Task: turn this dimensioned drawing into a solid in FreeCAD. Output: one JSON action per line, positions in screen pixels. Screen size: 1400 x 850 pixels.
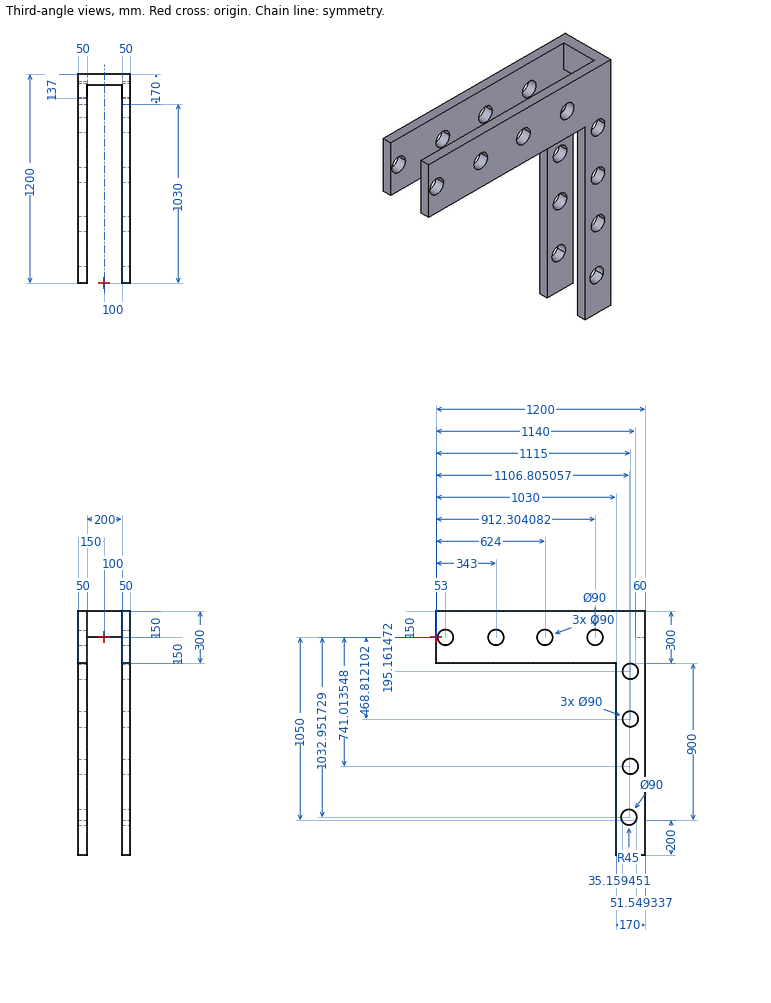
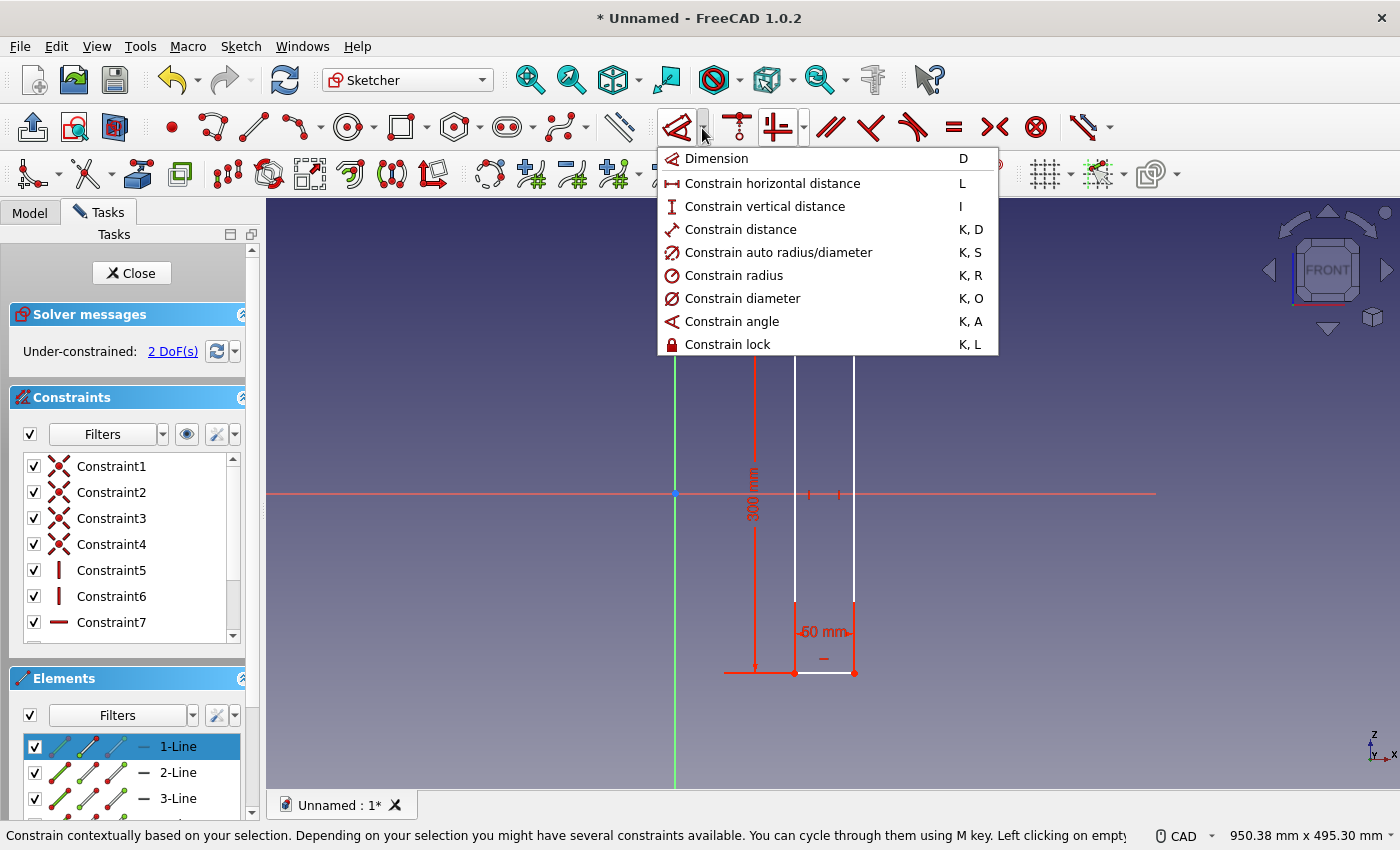
{"action": "left_click", "coordinate": [828, 184]}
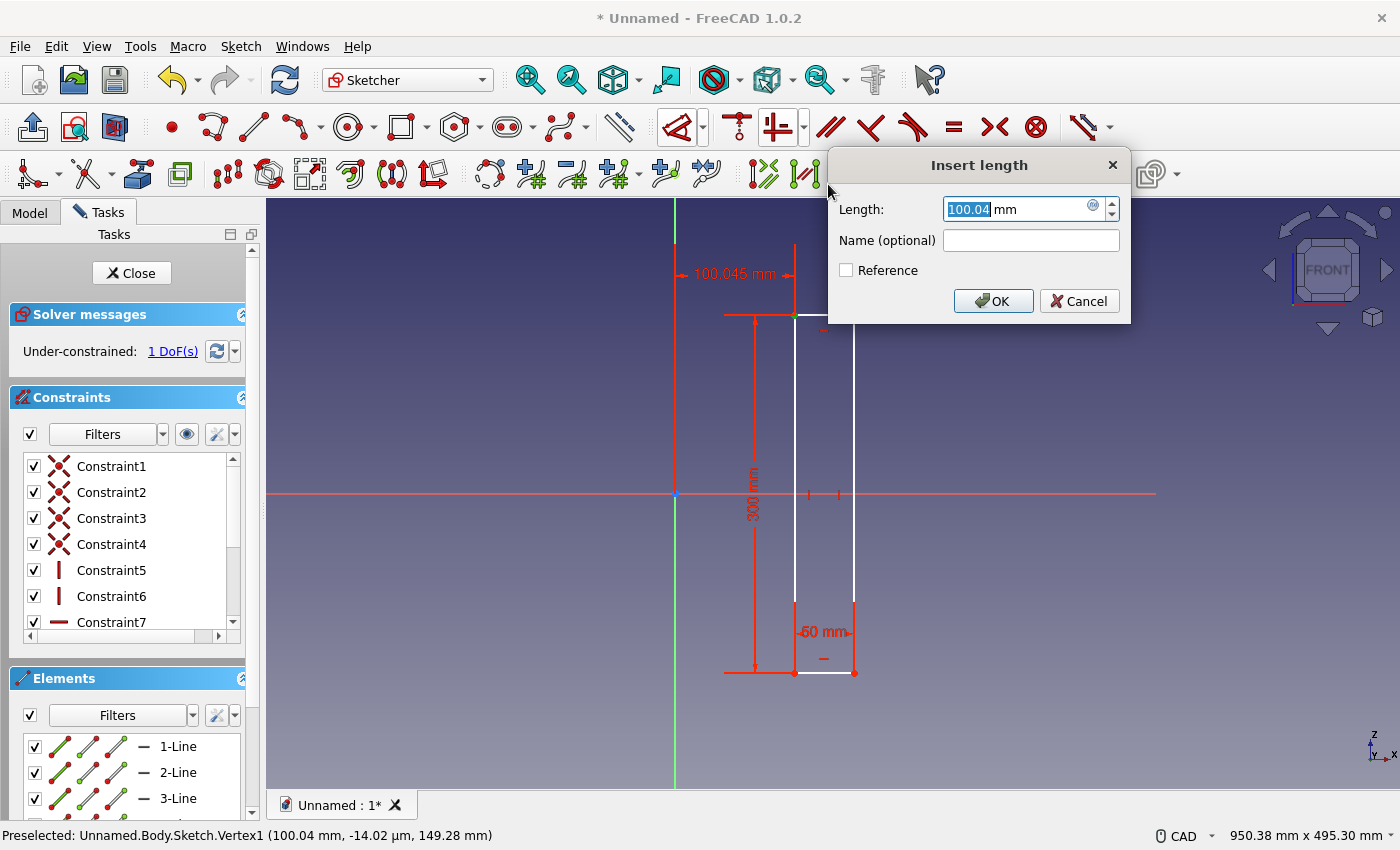
{"action": "type", "text": "100"}
{"action": "key", "text": "Return"}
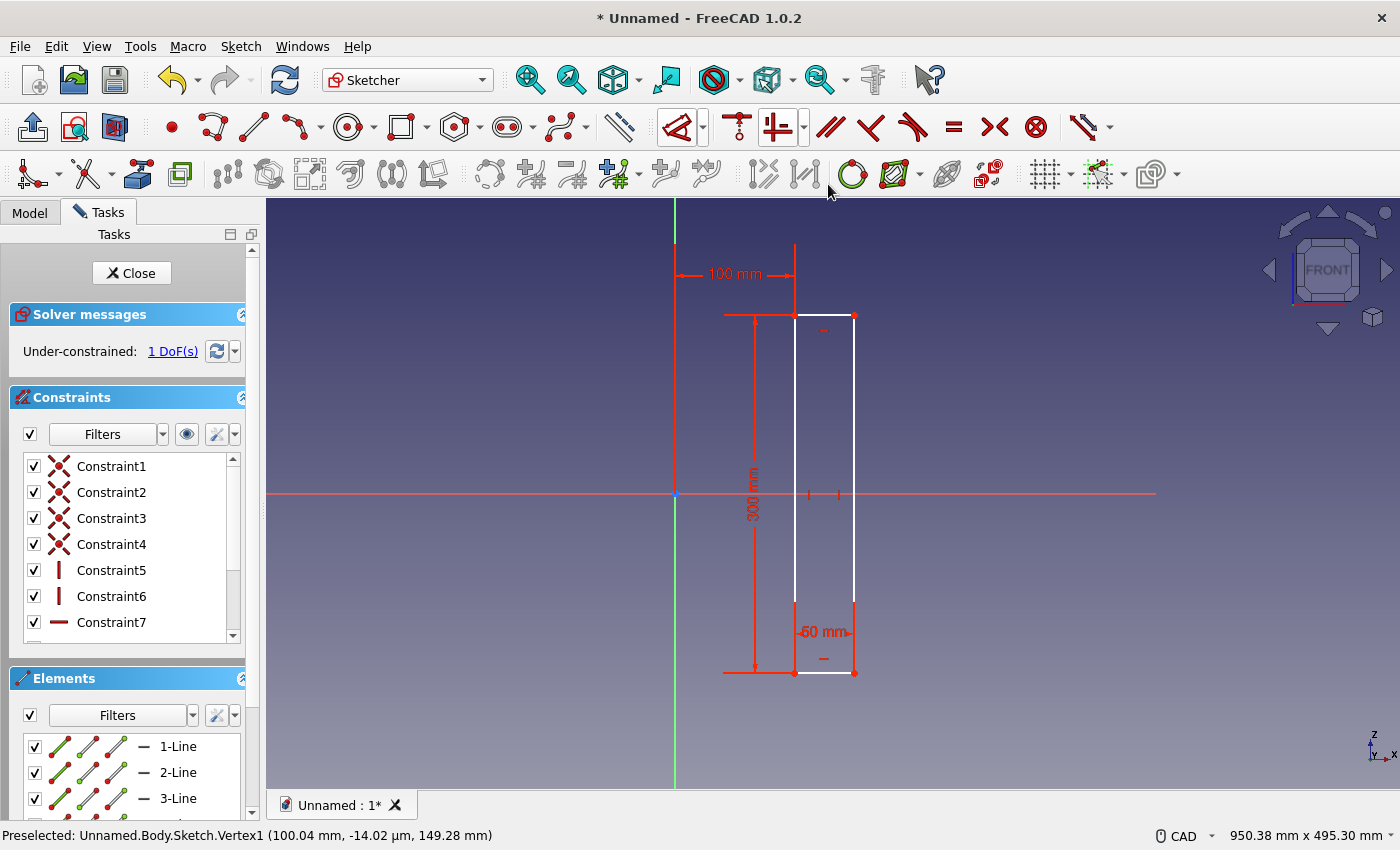
{"action": "left_click", "coordinate": [795, 315]}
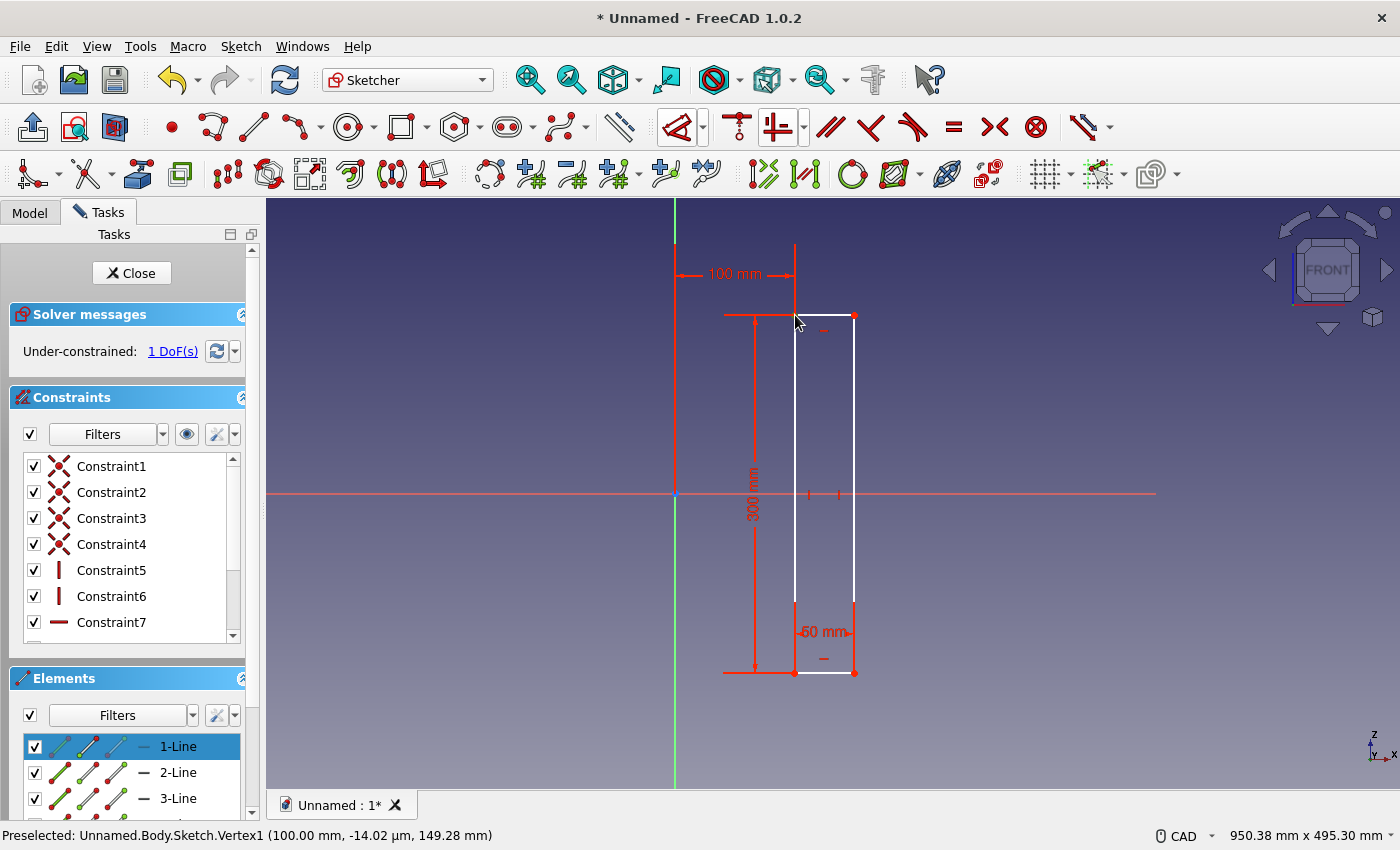
{"action": "key", "text": "i"}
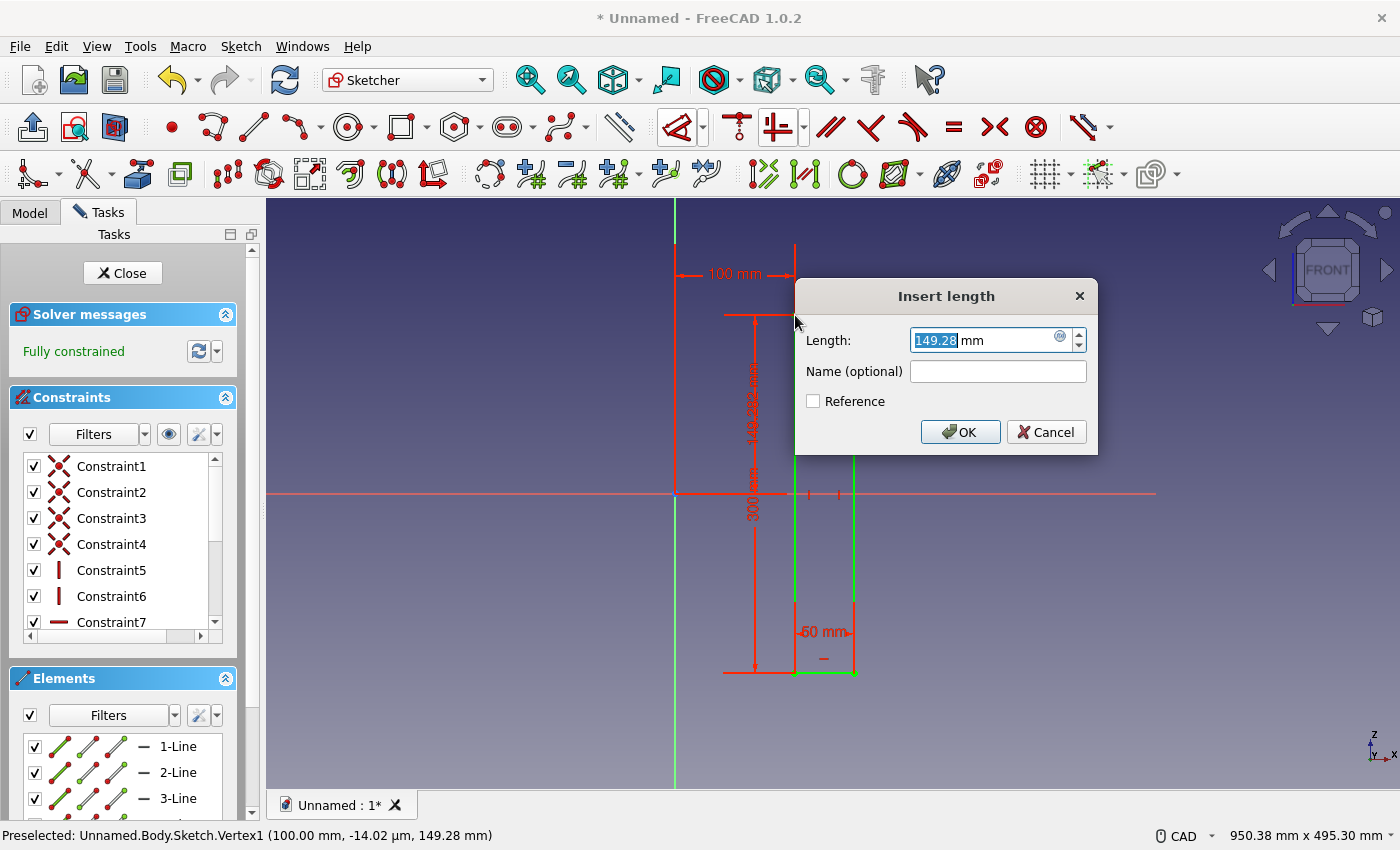
{"action": "type", "text": "150"}
{"action": "key", "text": "Return"}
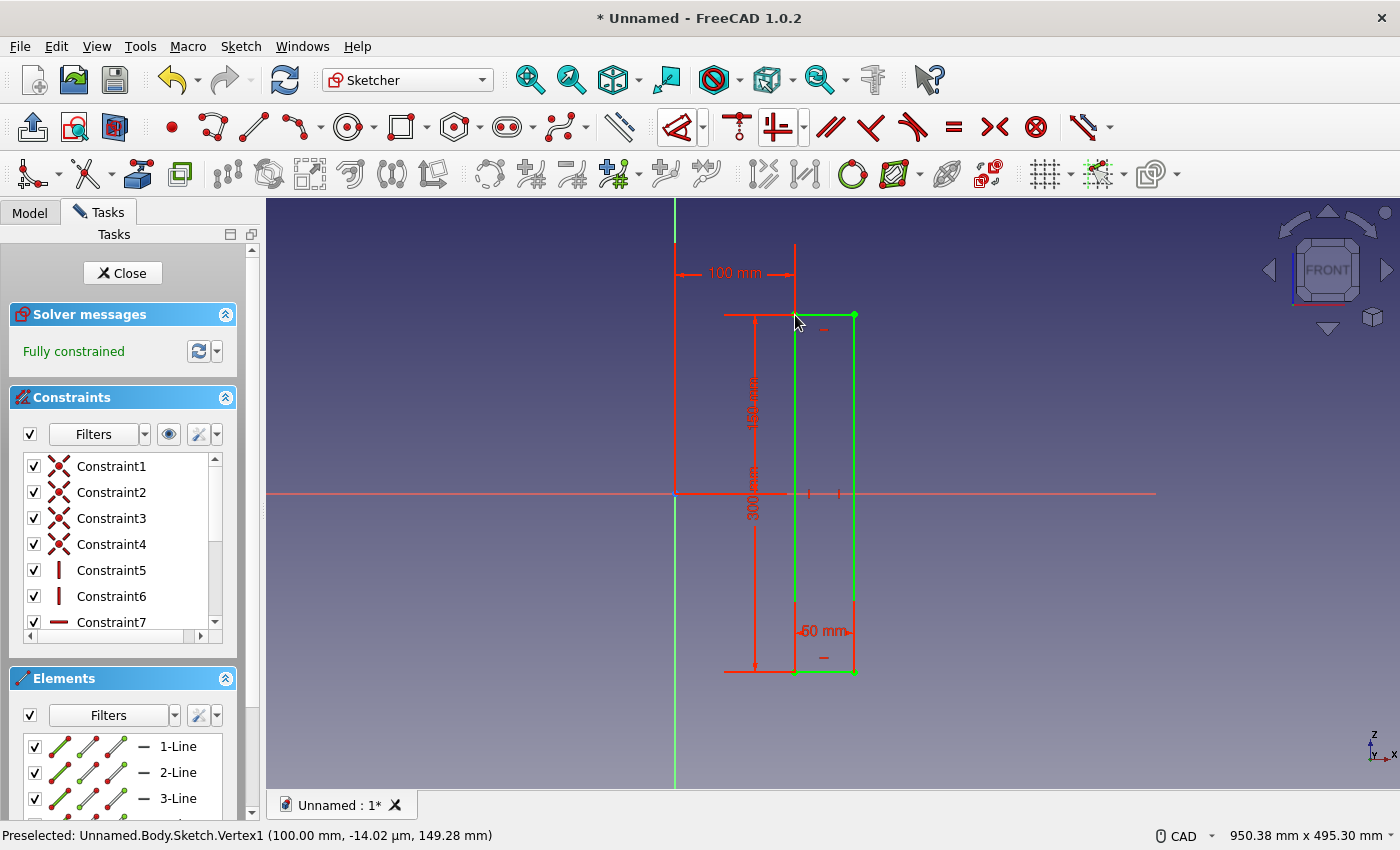
{"action": "left_click", "coordinate": [123, 273]}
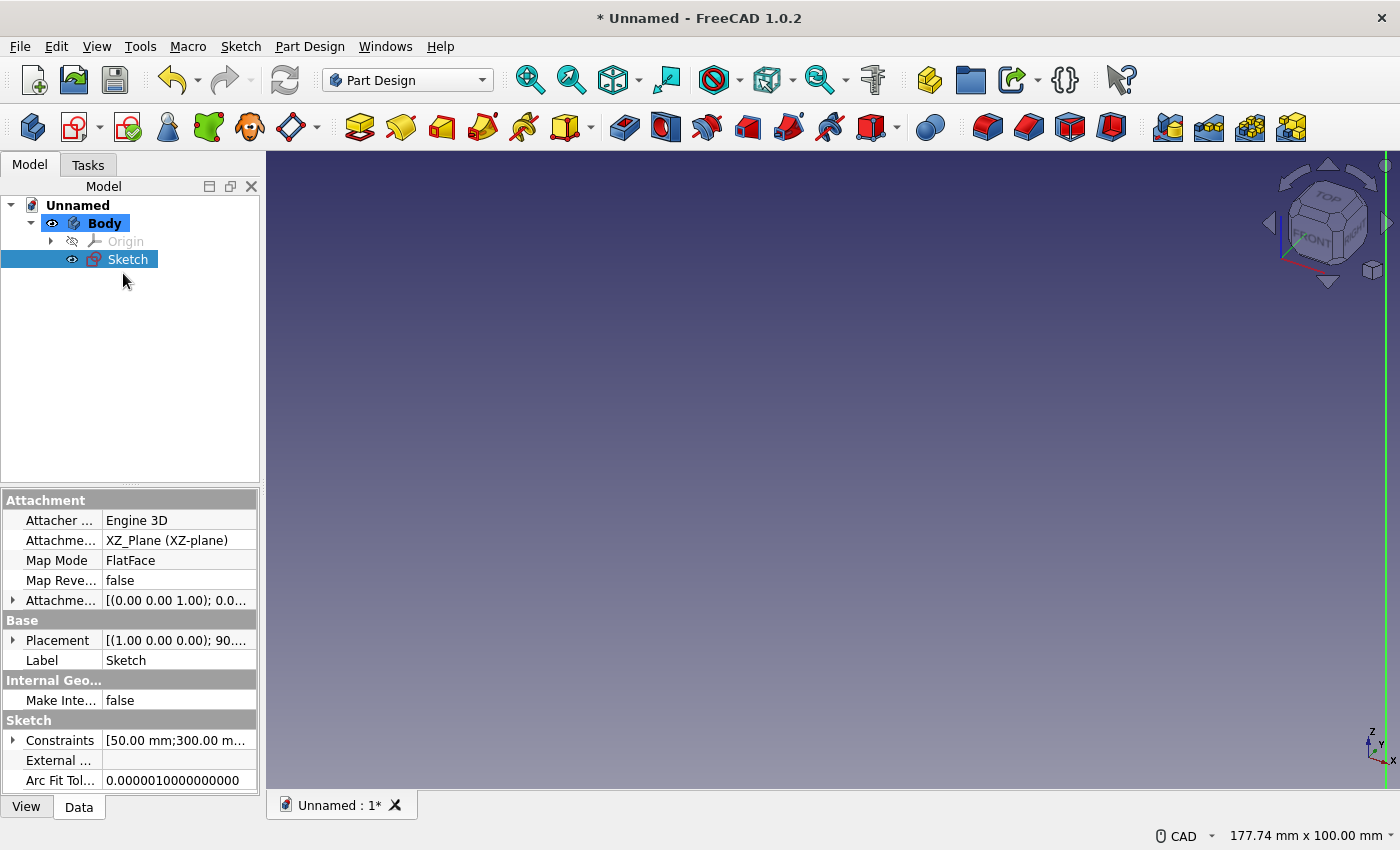
{"action": "left_click", "coordinate": [360, 128]}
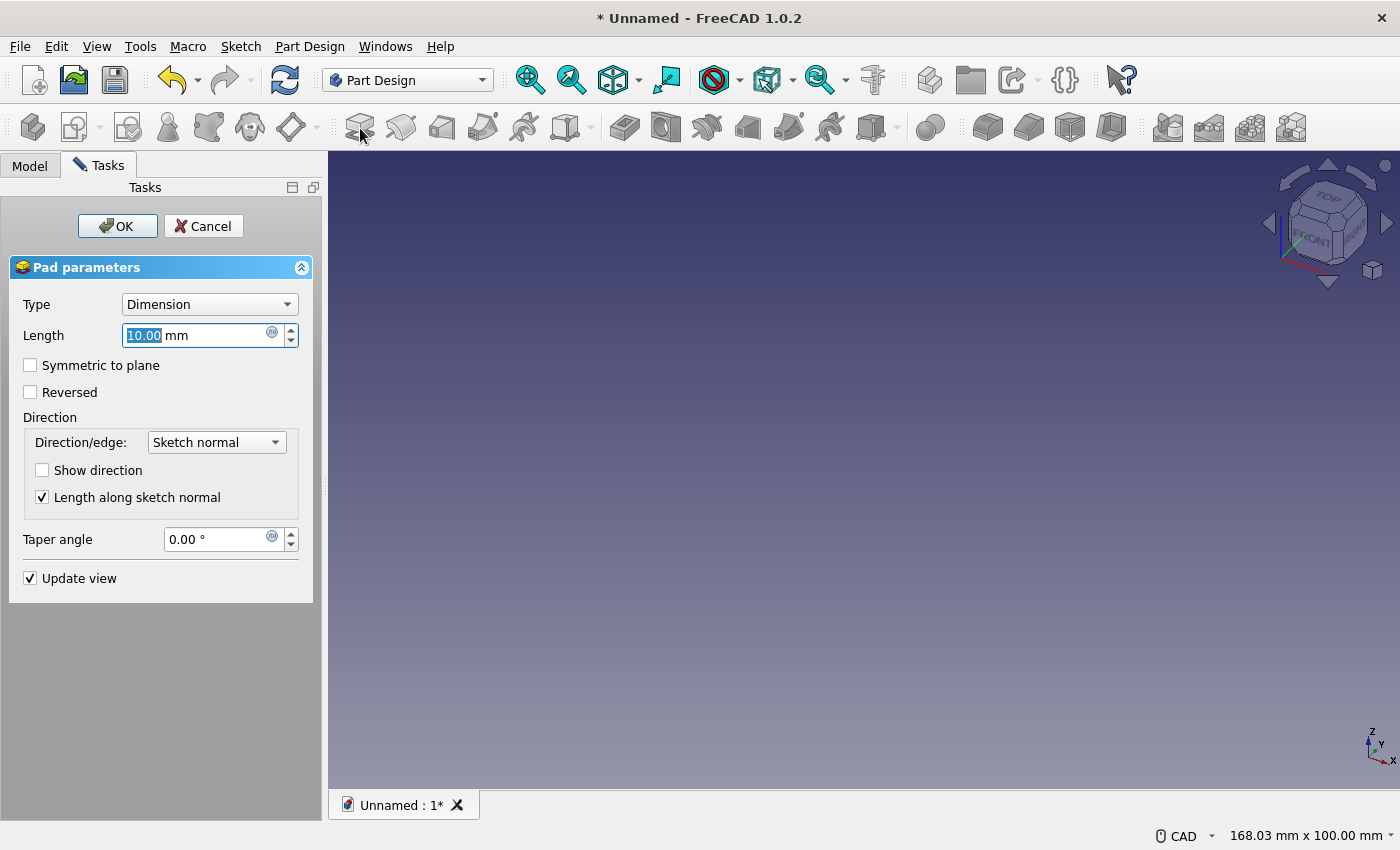
{"action": "type", "text": "1200"}
{"action": "key", "text": "Tab"}